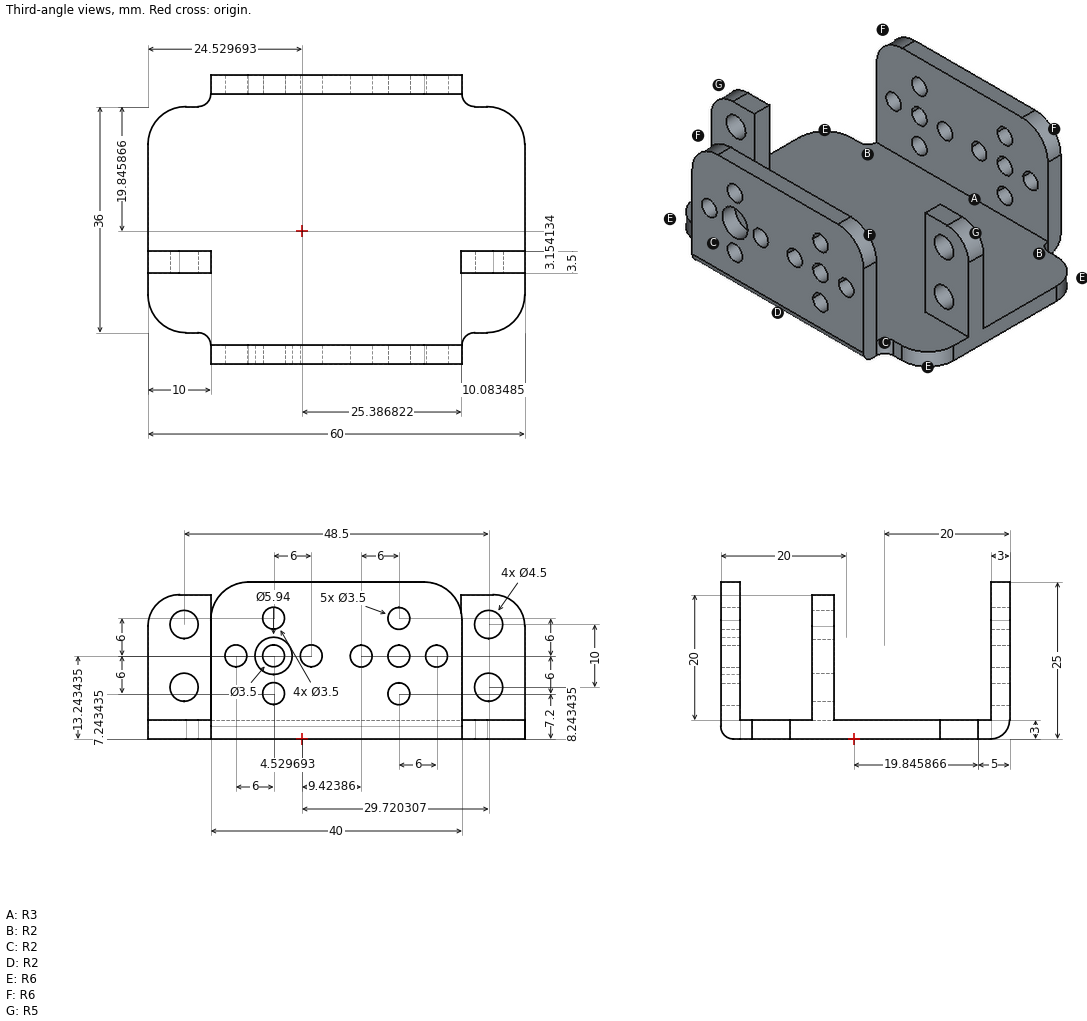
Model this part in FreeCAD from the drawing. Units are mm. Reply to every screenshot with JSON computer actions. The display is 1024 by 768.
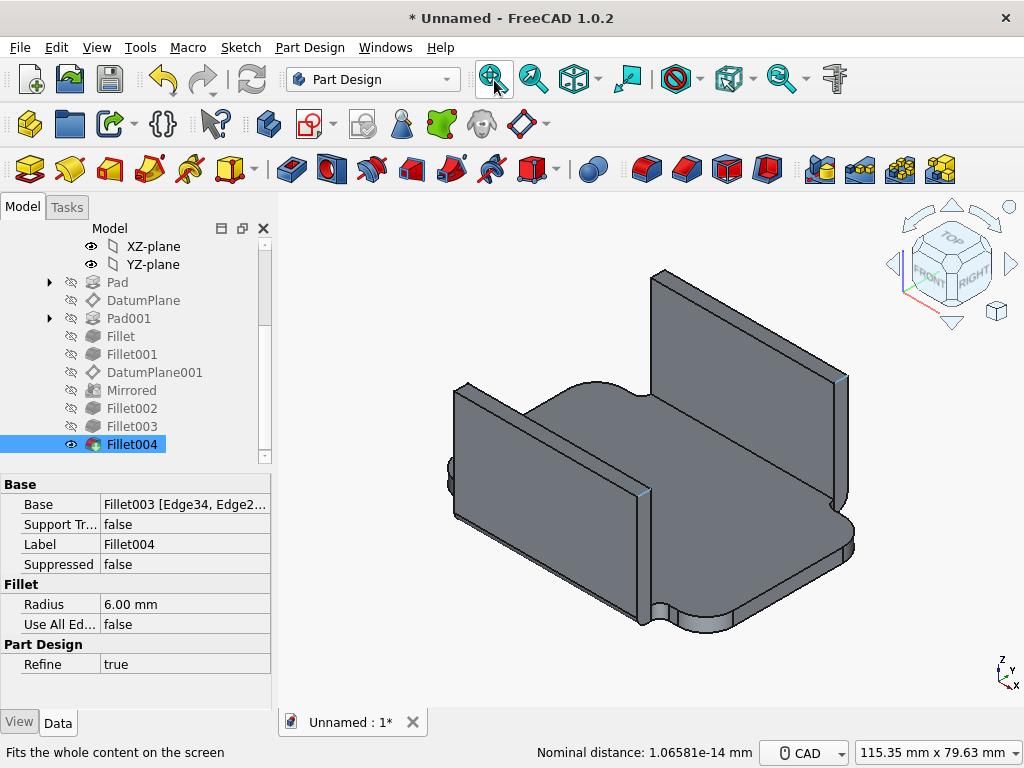
{"action": "key", "text": "2"}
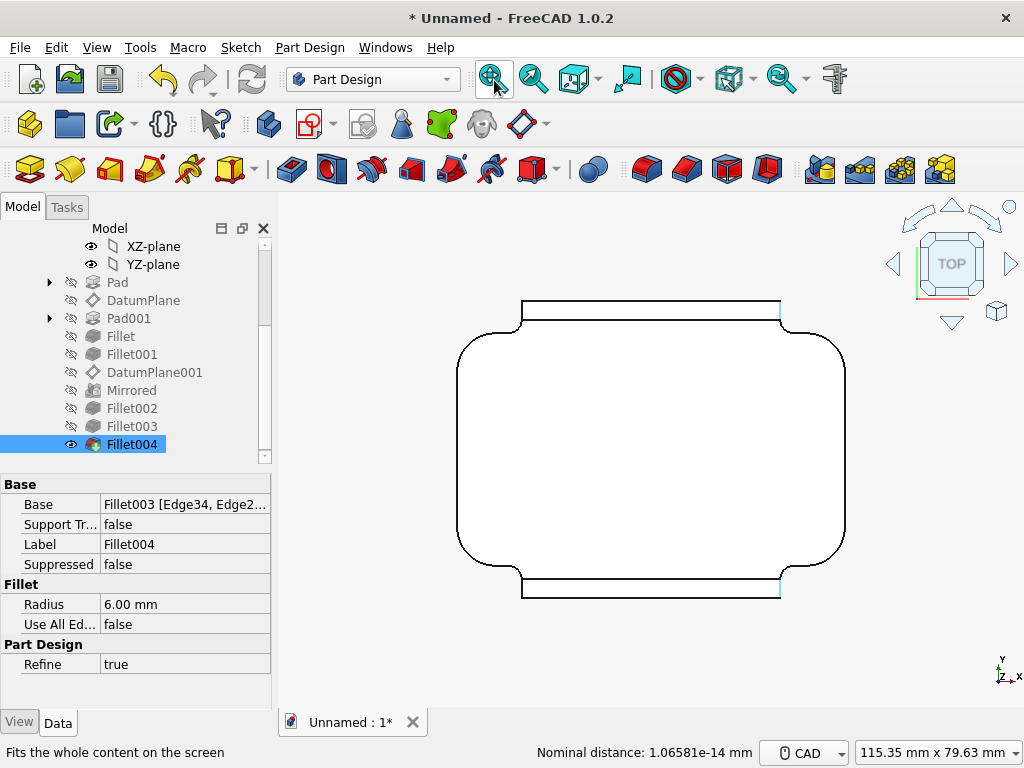
{"action": "left_click", "coordinate": [522, 309], "text": "ctrl"}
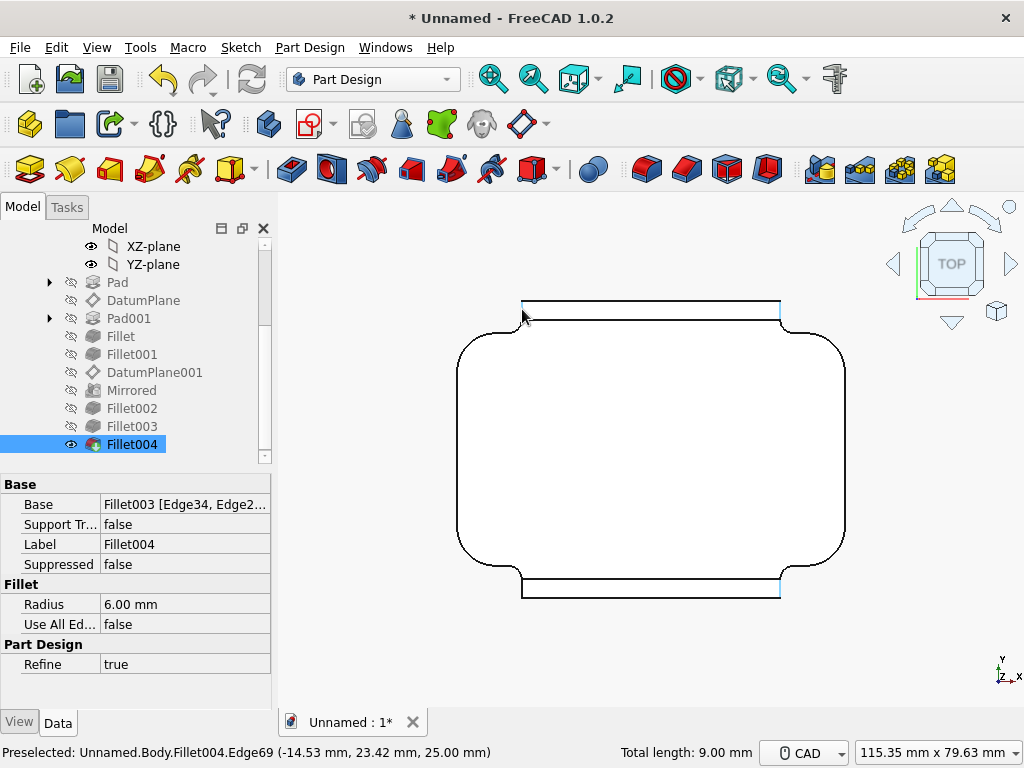
{"action": "left_click", "coordinate": [522, 588], "text": "ctrl"}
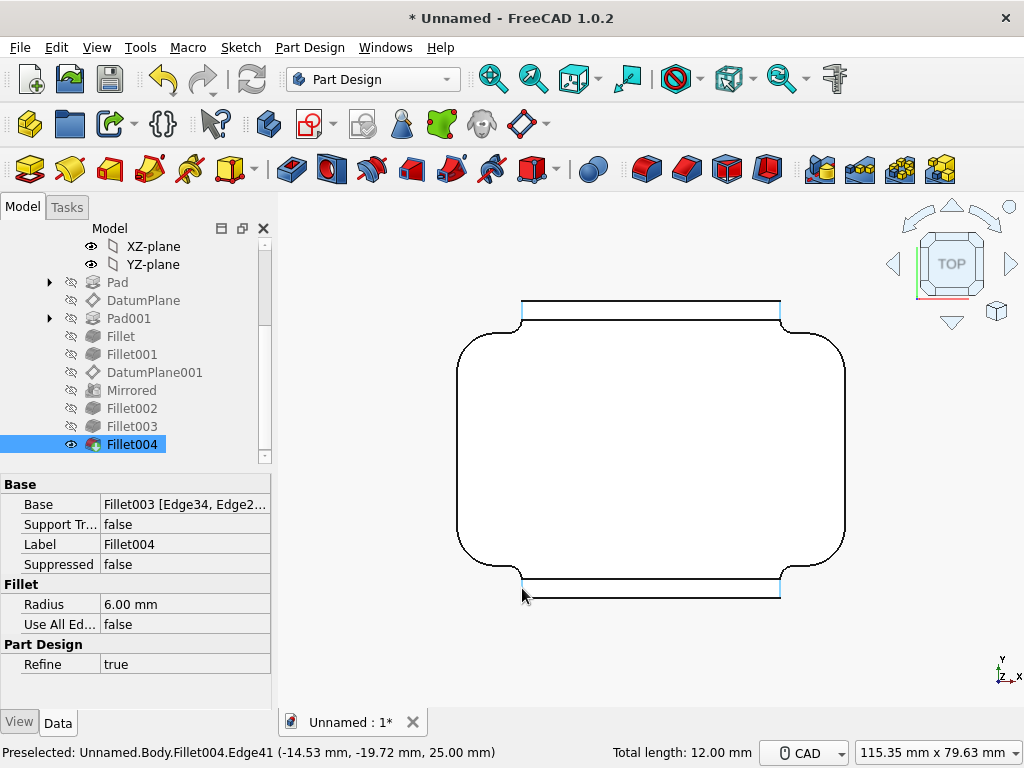
{"action": "left_click", "coordinate": [648, 170]}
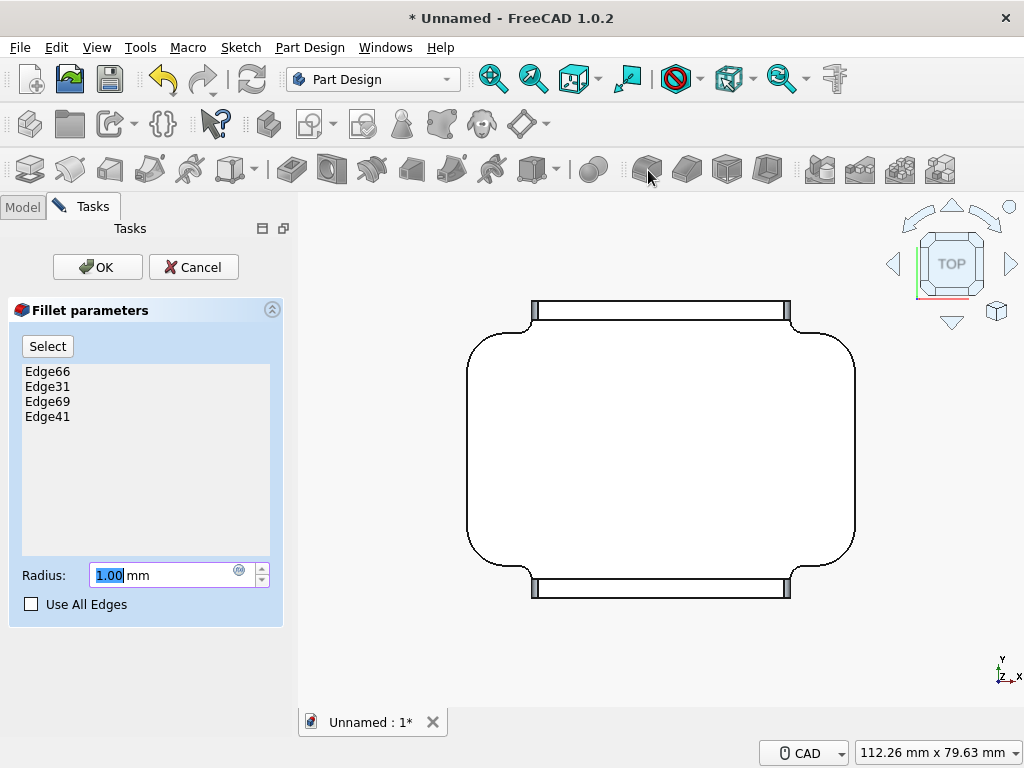
{"action": "type", "text": "6"}
{"action": "key", "text": "Tab"}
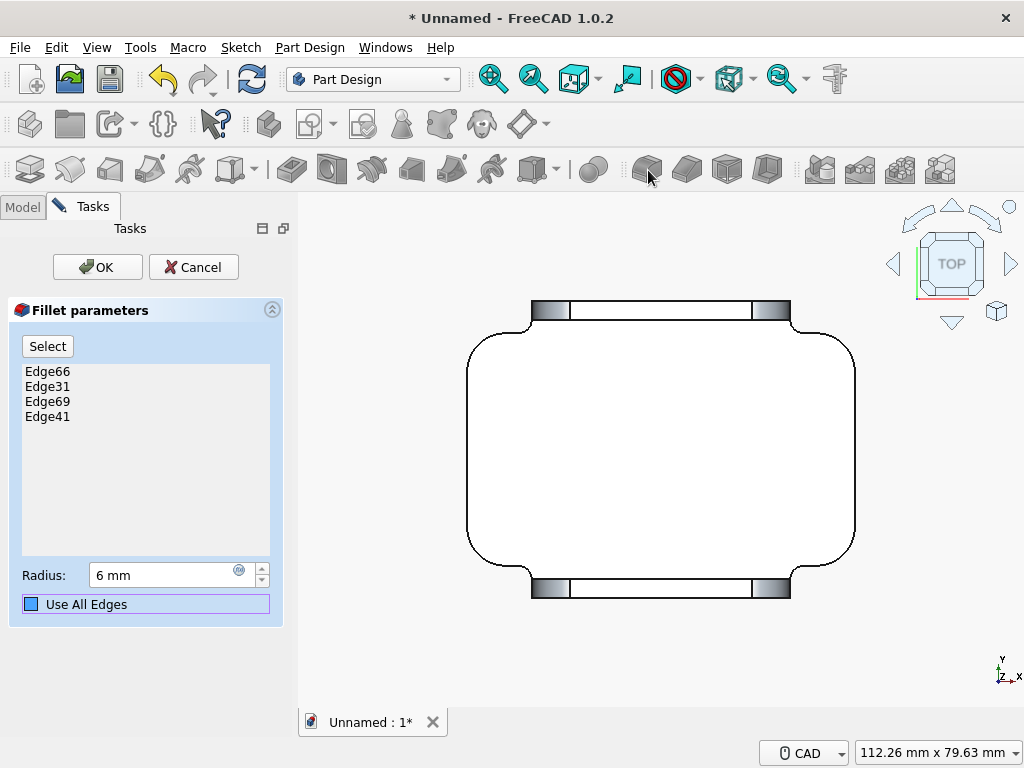
{"action": "left_click", "coordinate": [98, 267]}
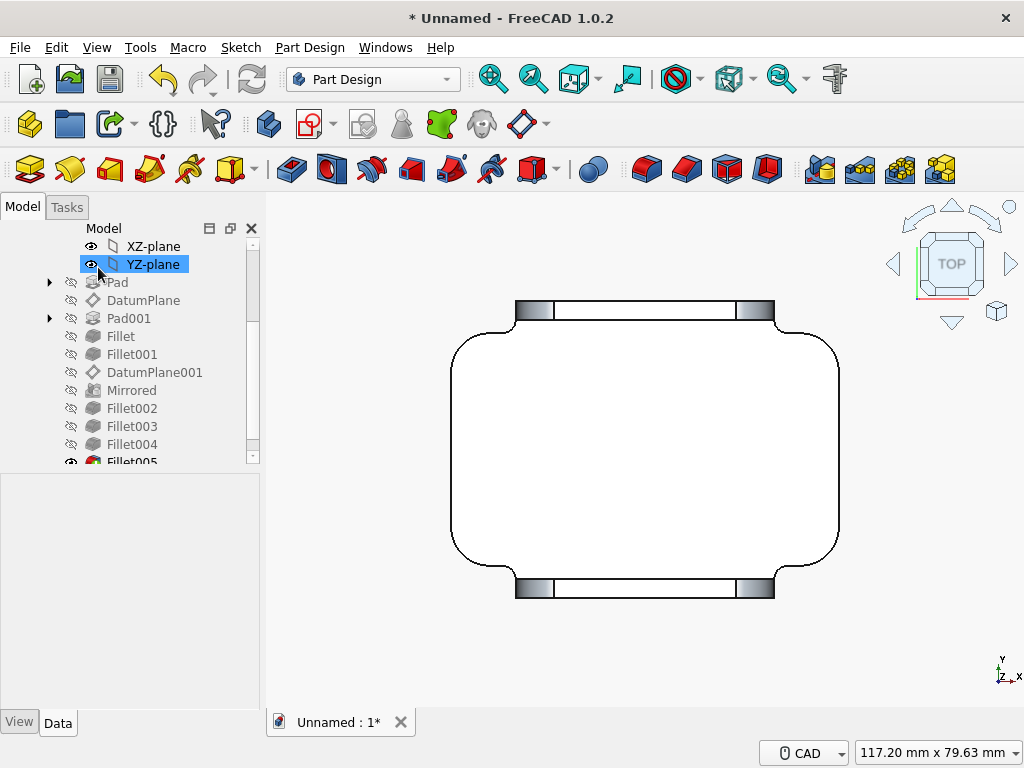
{"action": "key", "text": "4"}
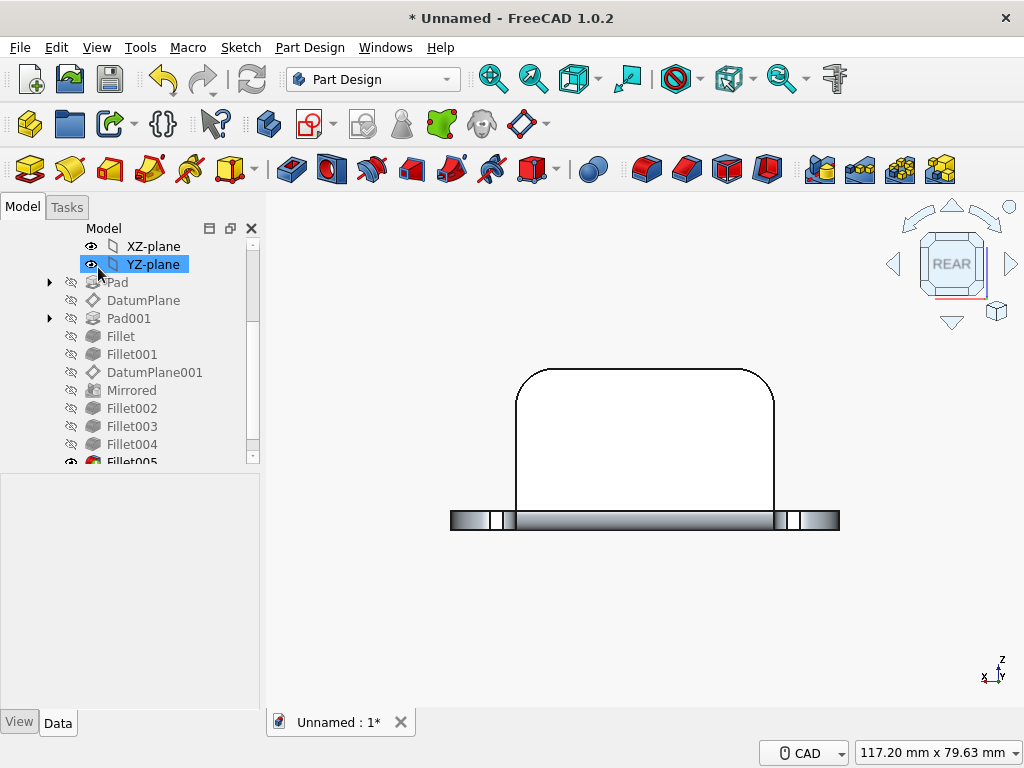
{"action": "left_click", "coordinate": [608, 439]}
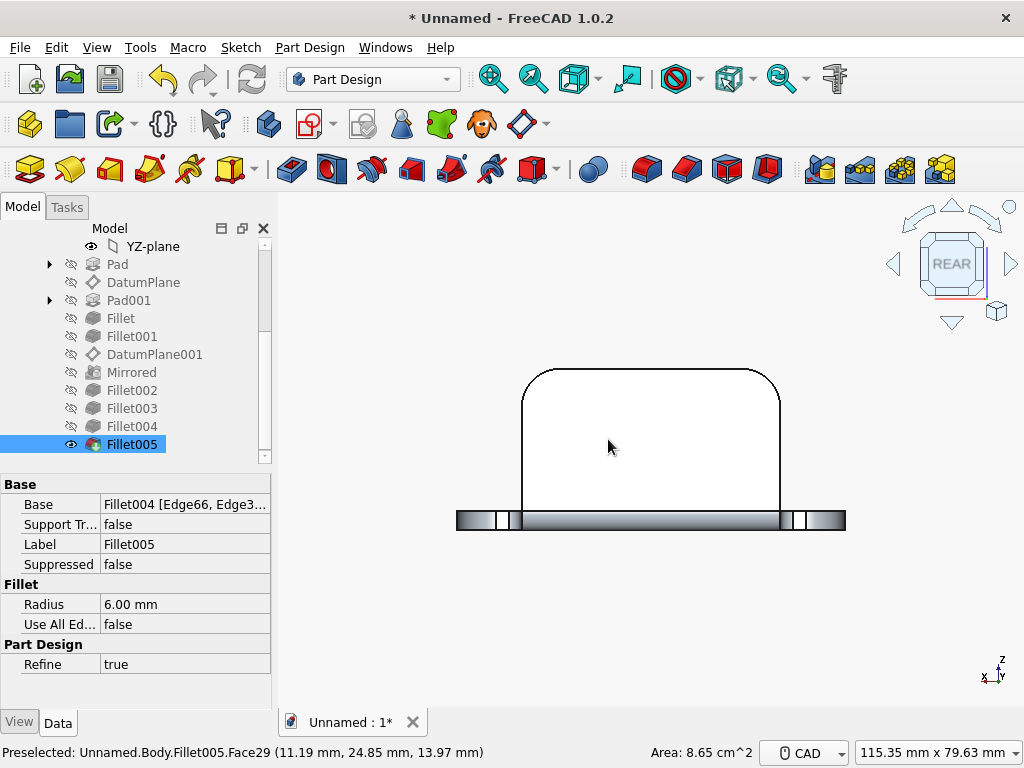
{"action": "left_click", "coordinate": [310, 124]}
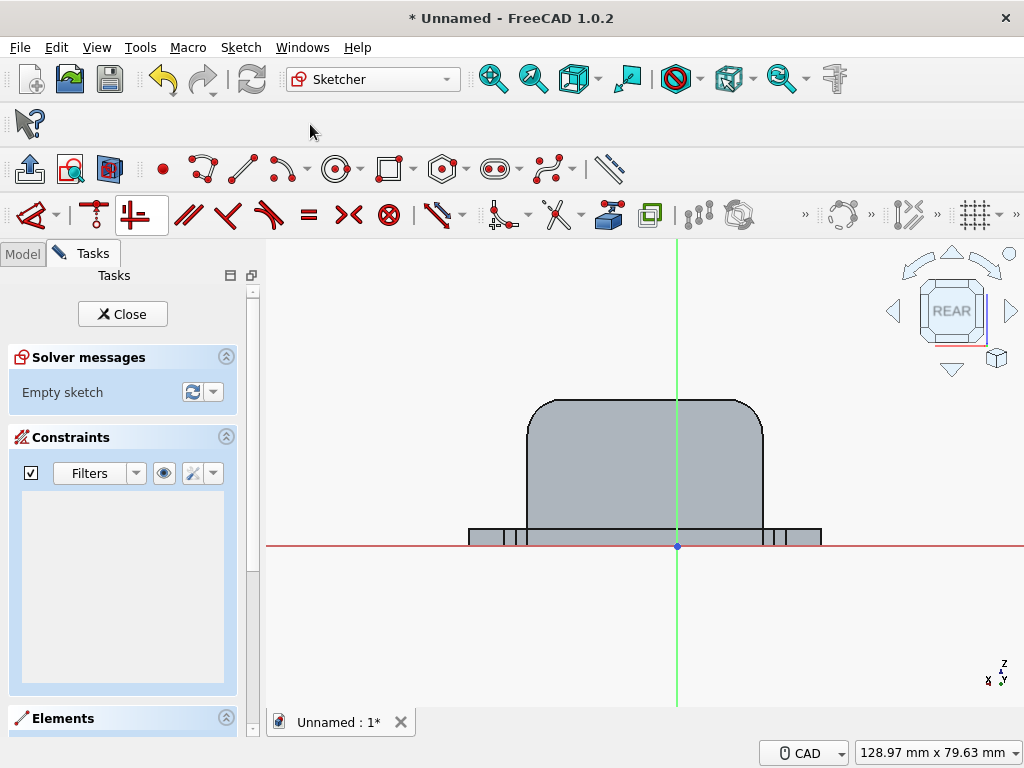
{"action": "scroll", "coordinate": [636, 495], "scroll_direction": "up", "scroll_amount": 4}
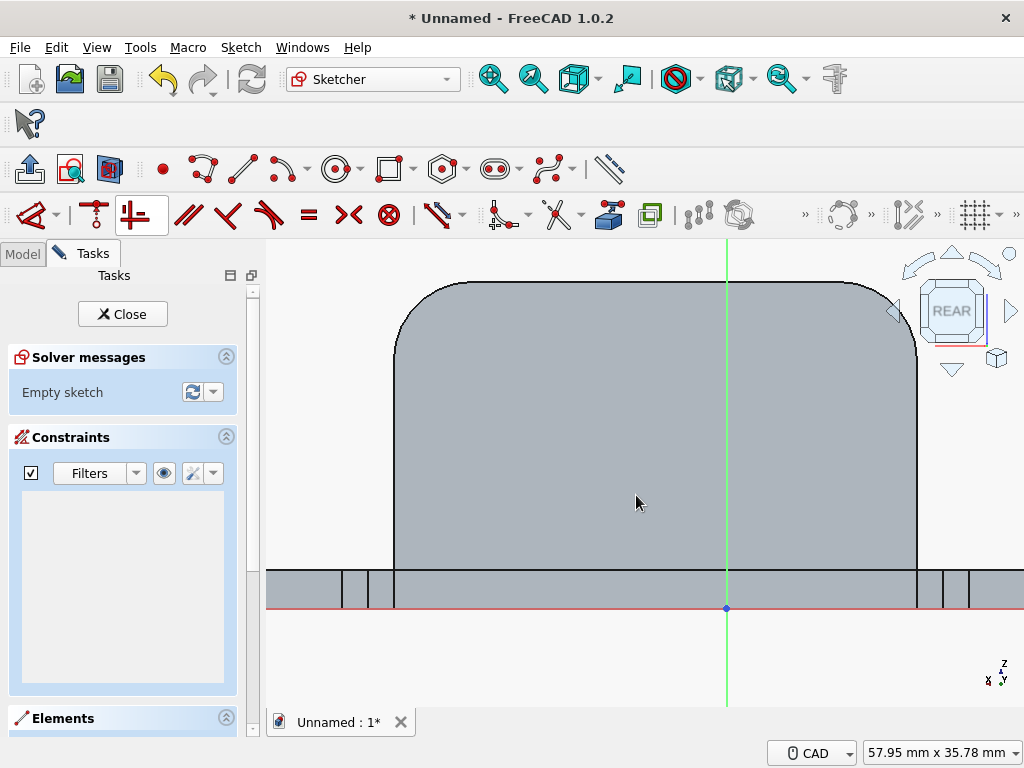
{"action": "left_click", "coordinate": [336, 170]}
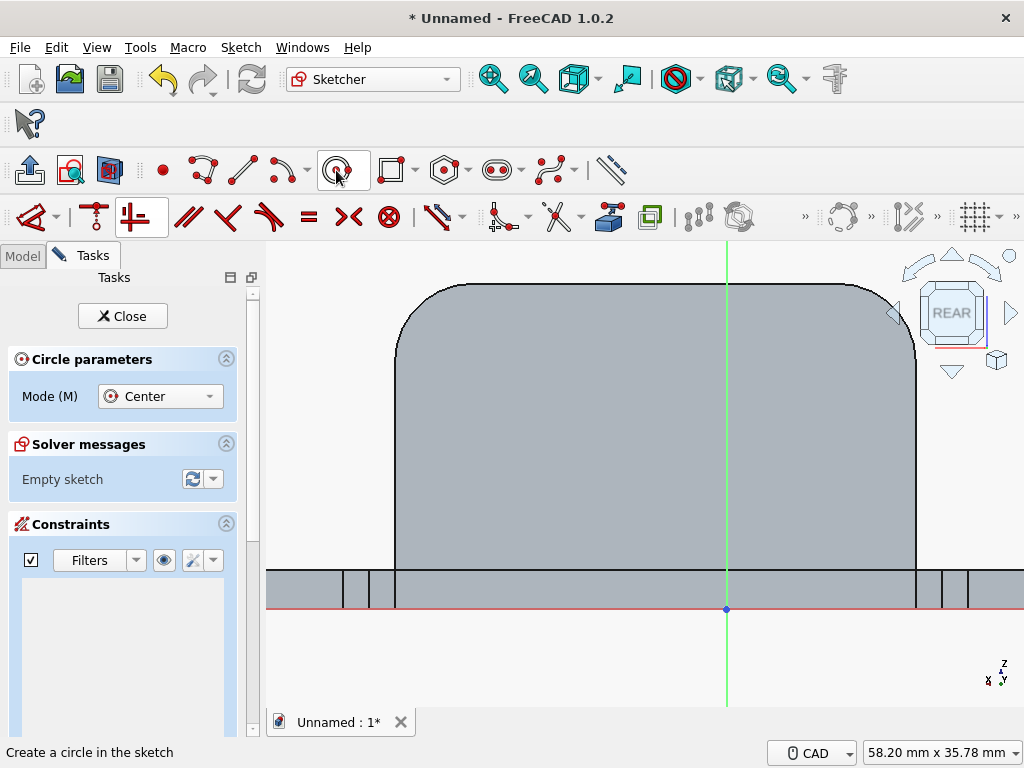
{"action": "left_click", "coordinate": [526, 359]}
{"action": "left_click", "coordinate": [542, 343]}